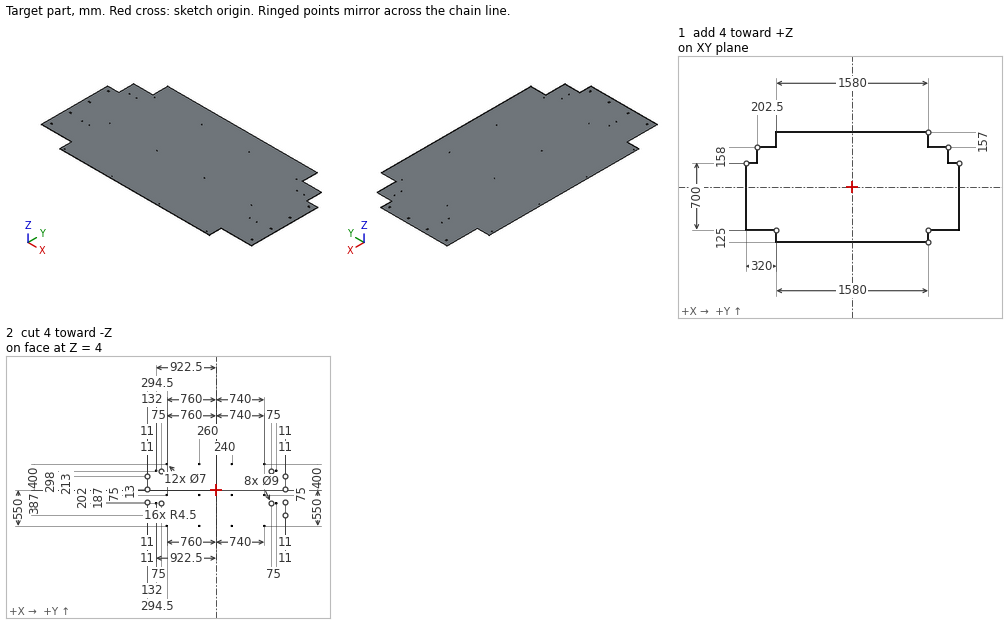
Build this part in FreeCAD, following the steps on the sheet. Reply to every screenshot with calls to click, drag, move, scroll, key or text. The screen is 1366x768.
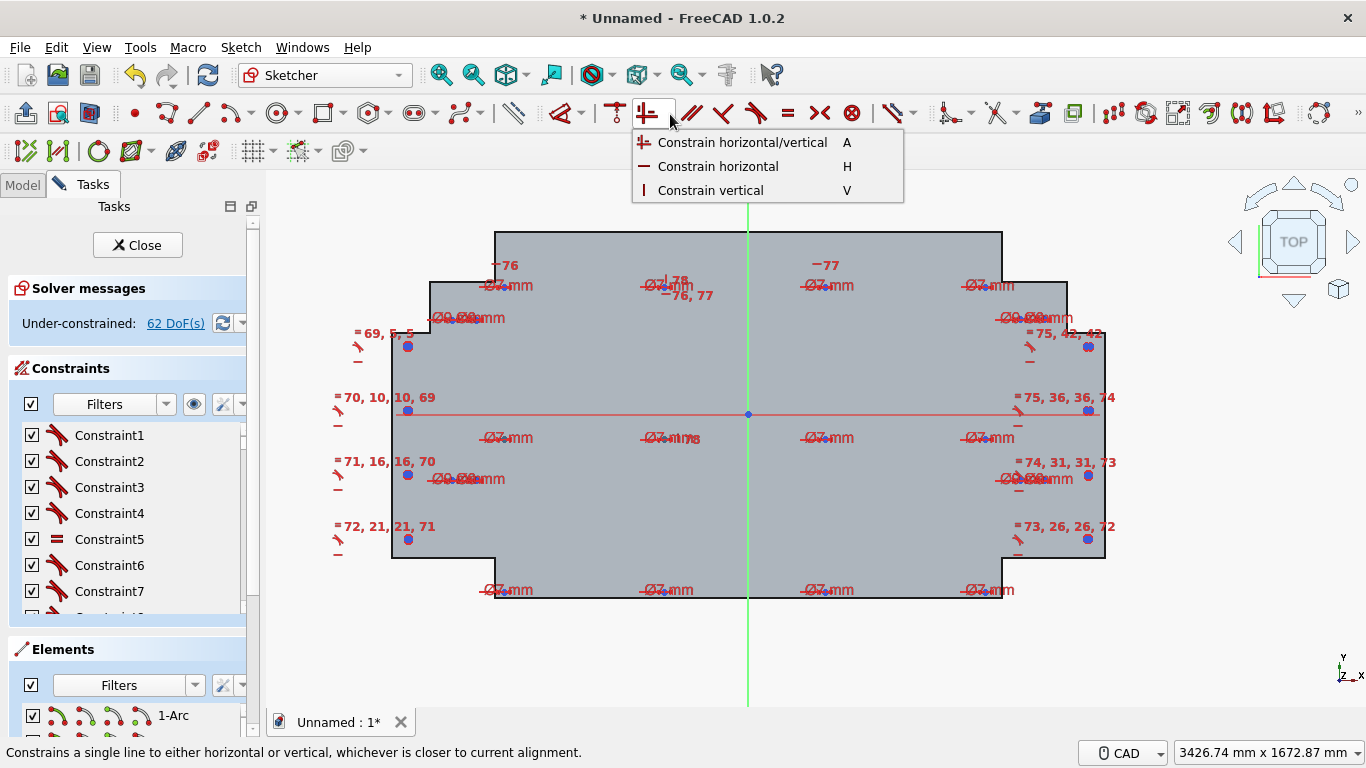
click(768, 166)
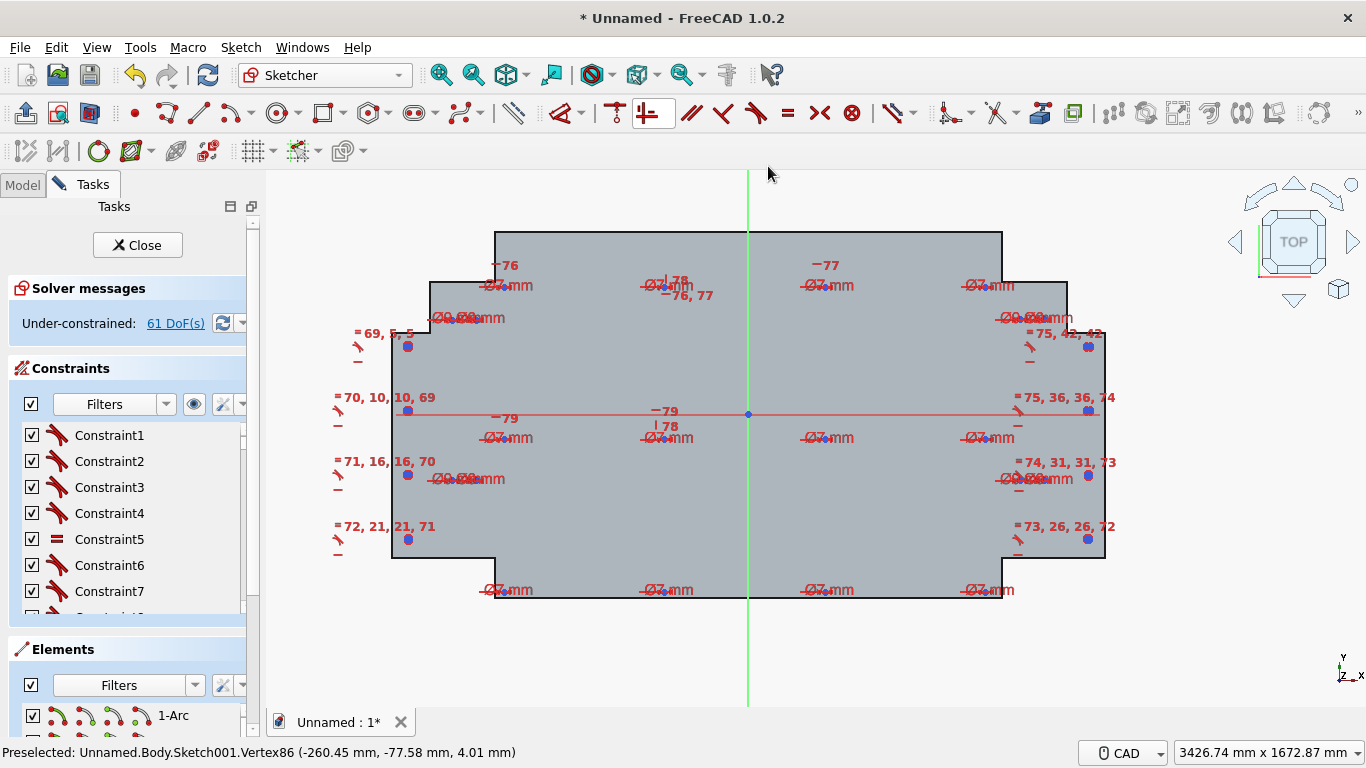
click(825, 287)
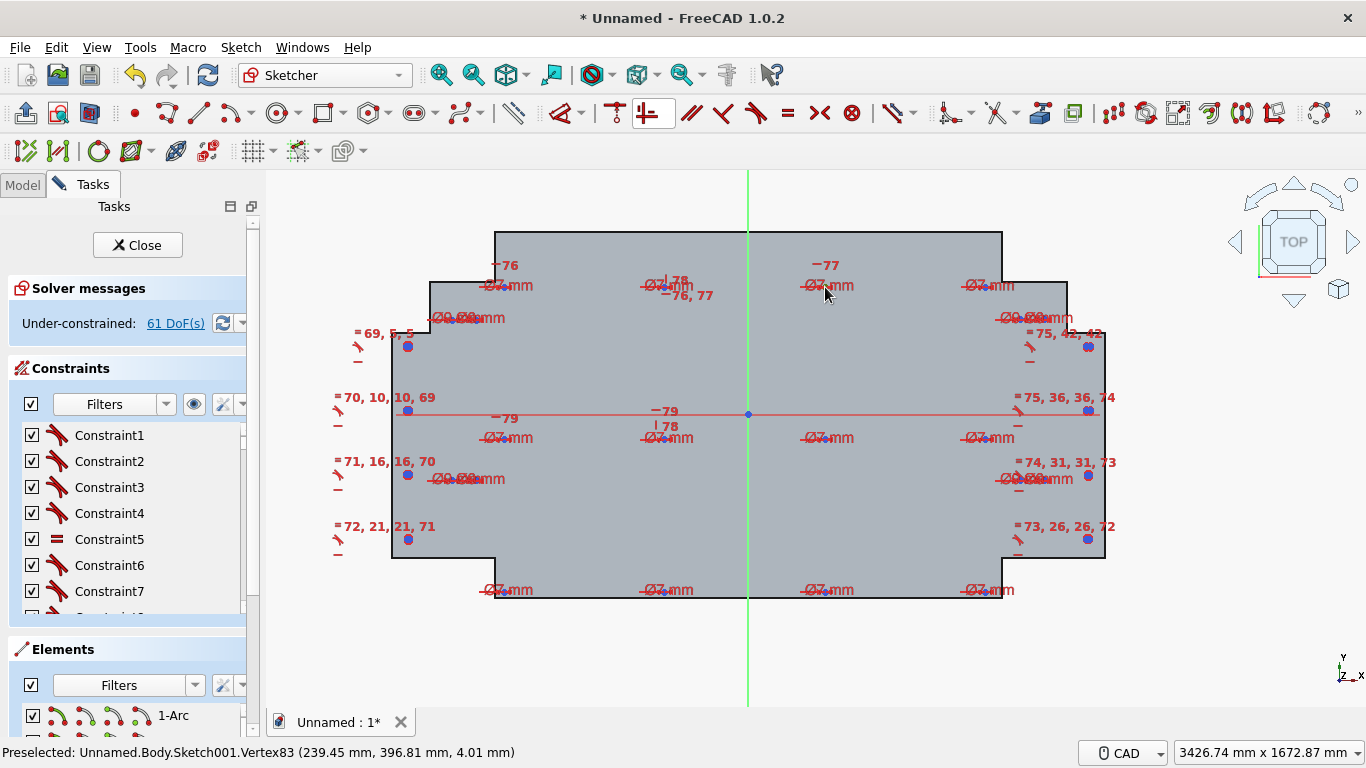
click(825, 440)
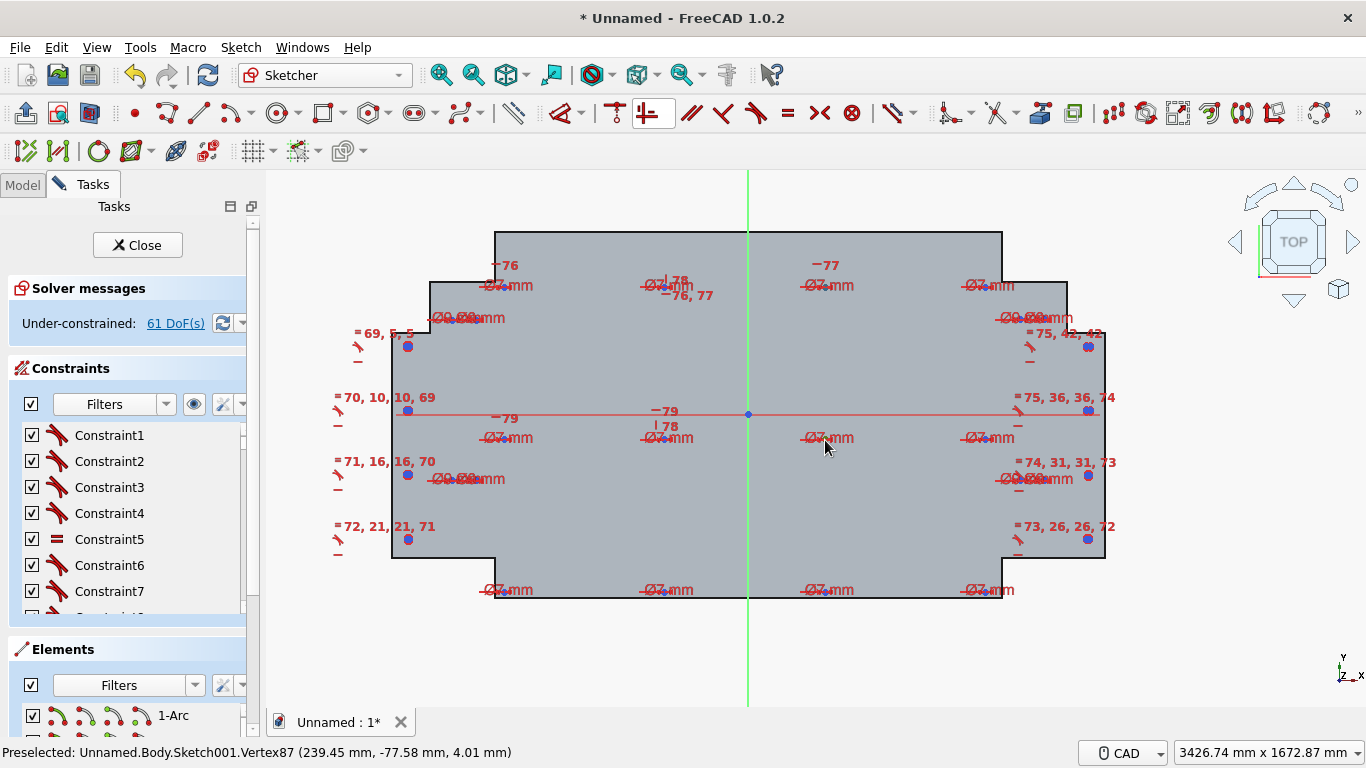
click(670, 114)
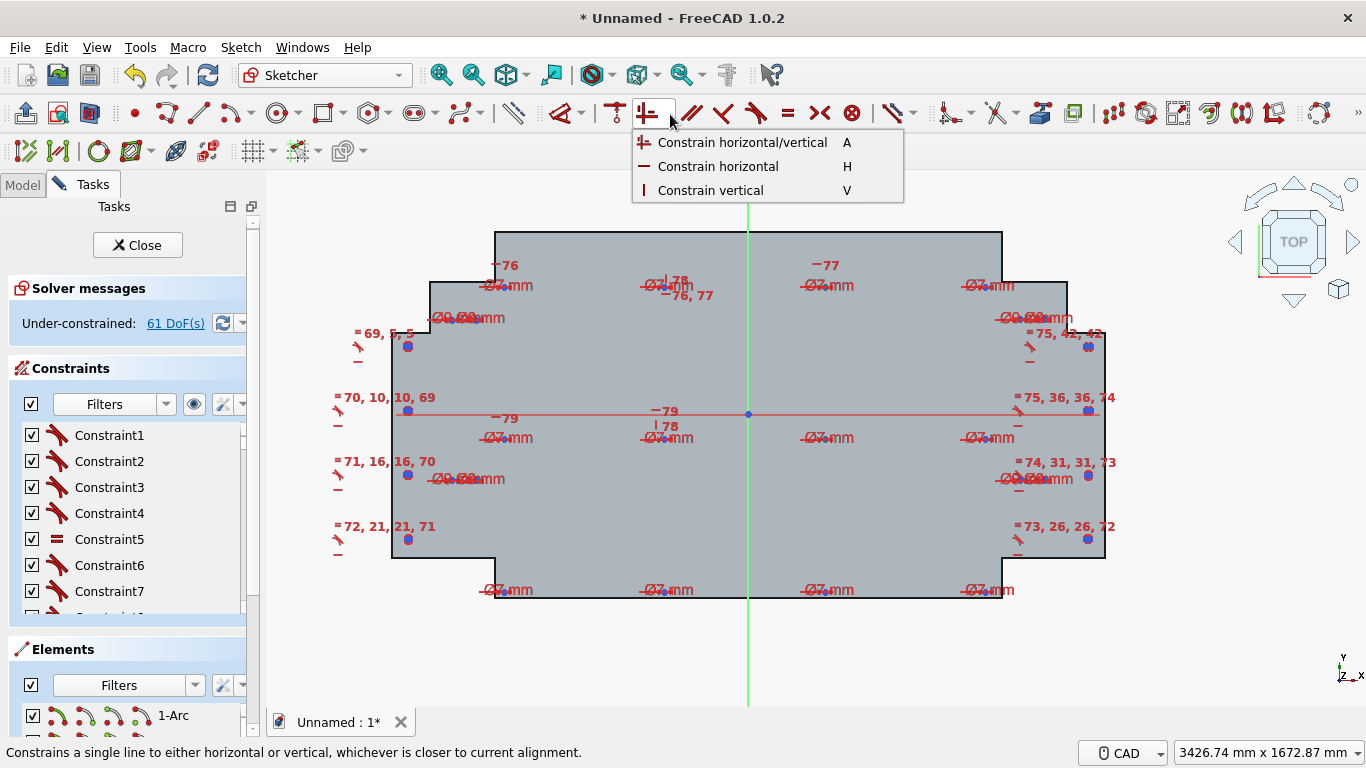
click(768, 190)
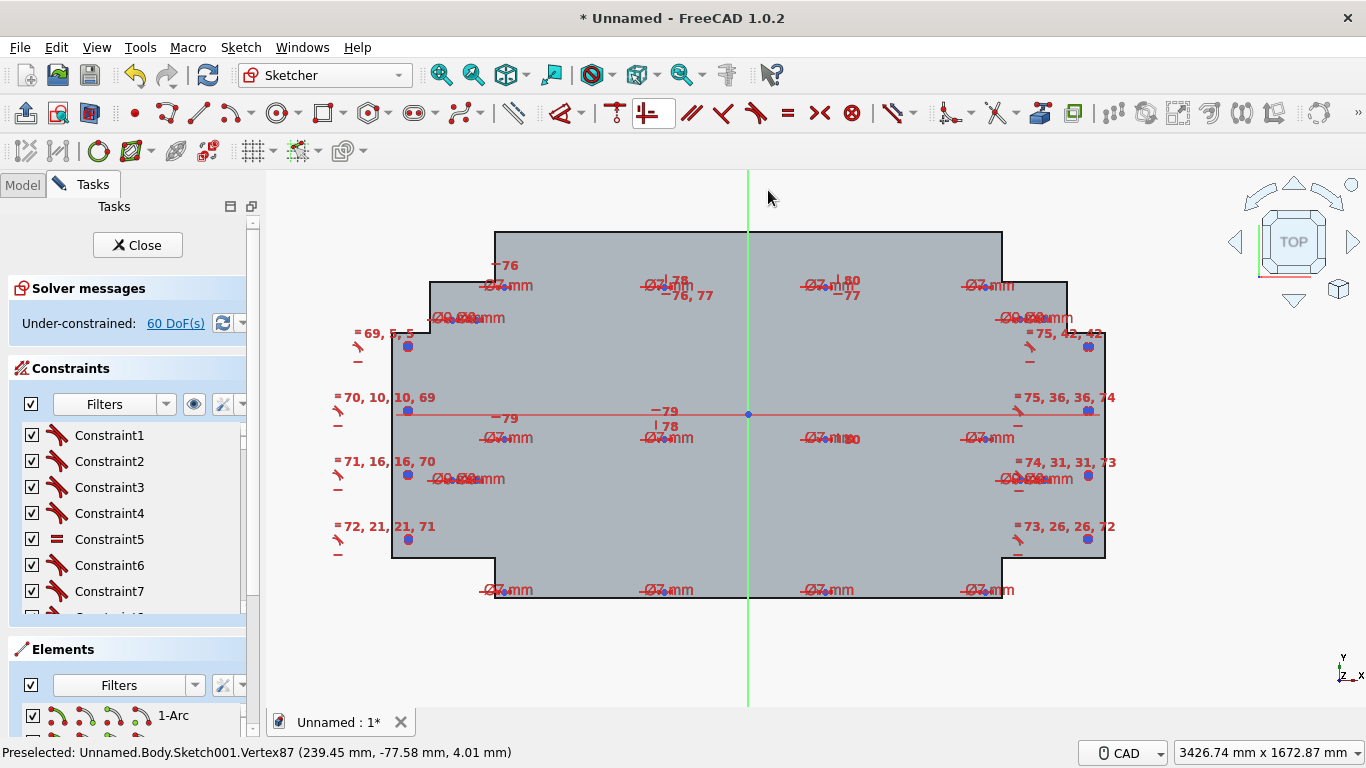
click(665, 440)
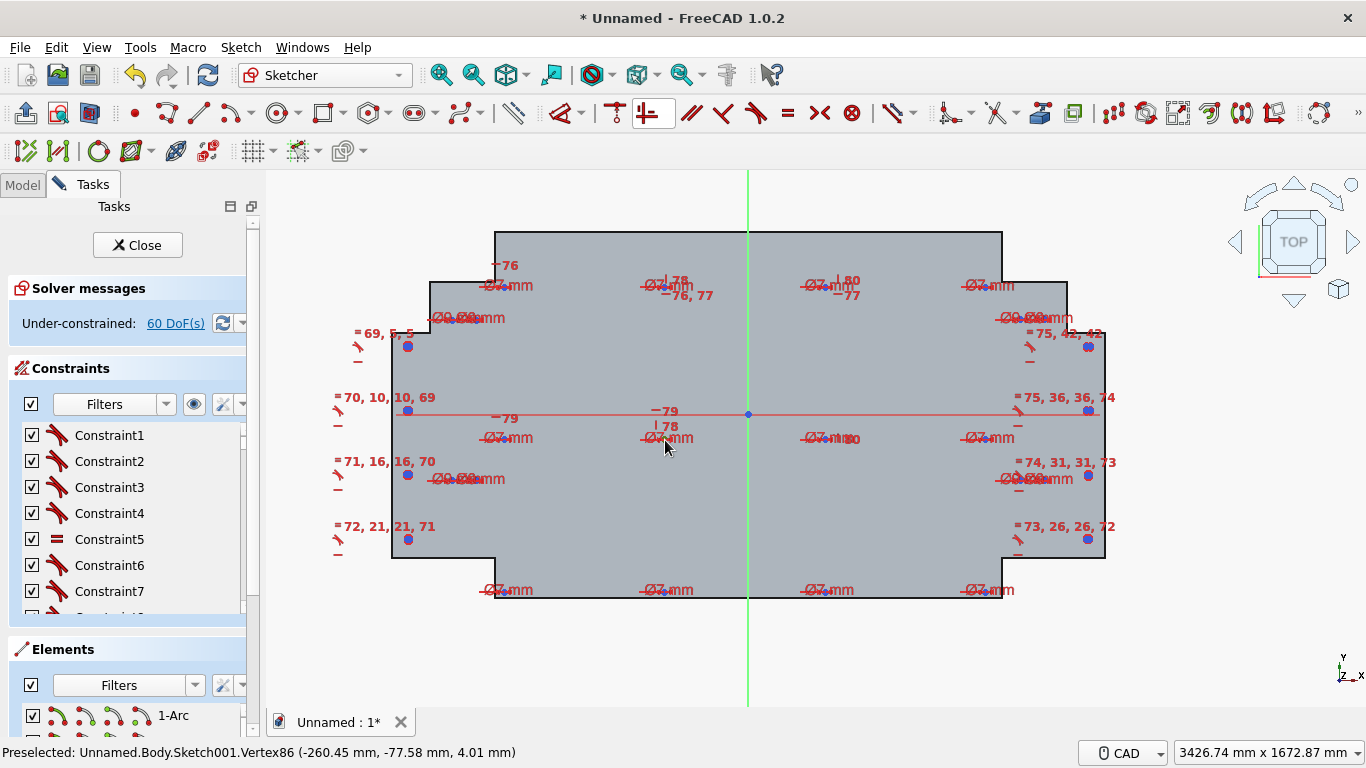
click(825, 440)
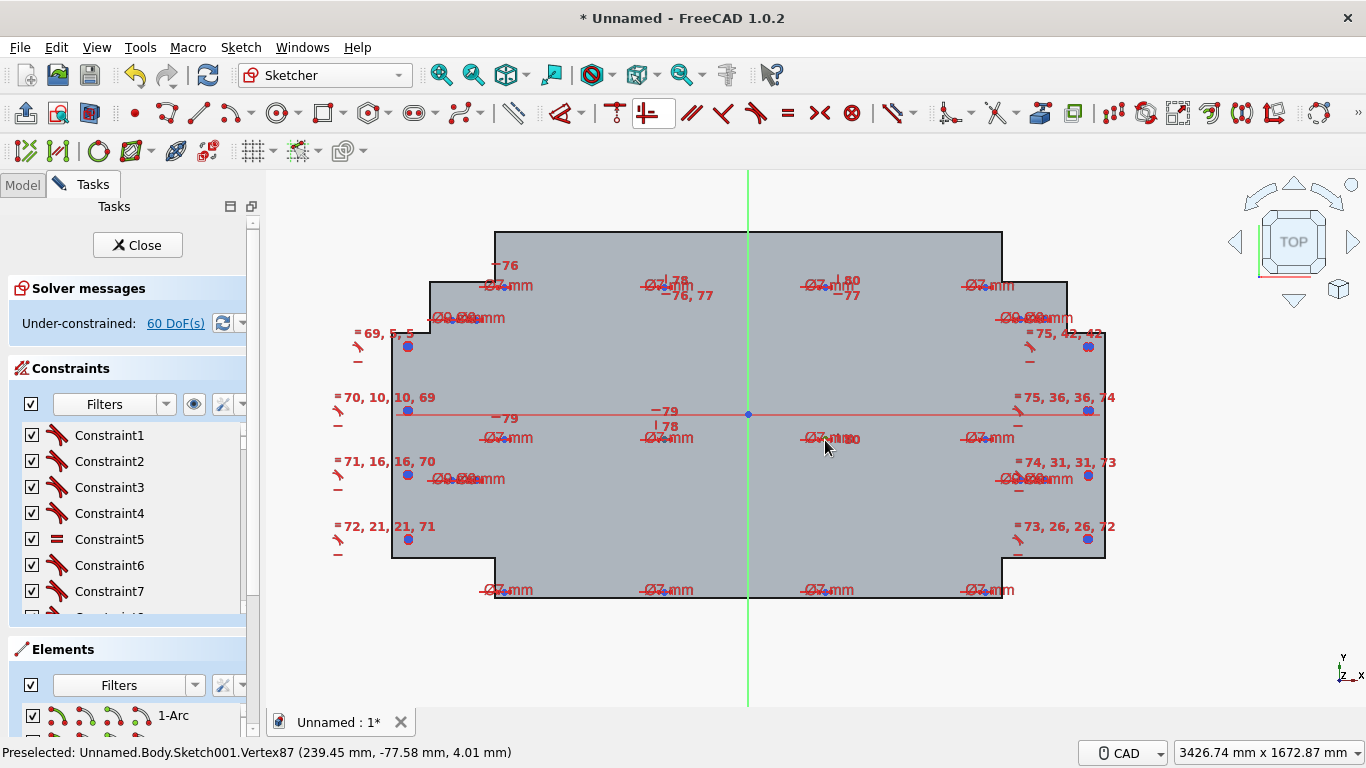
click(670, 114)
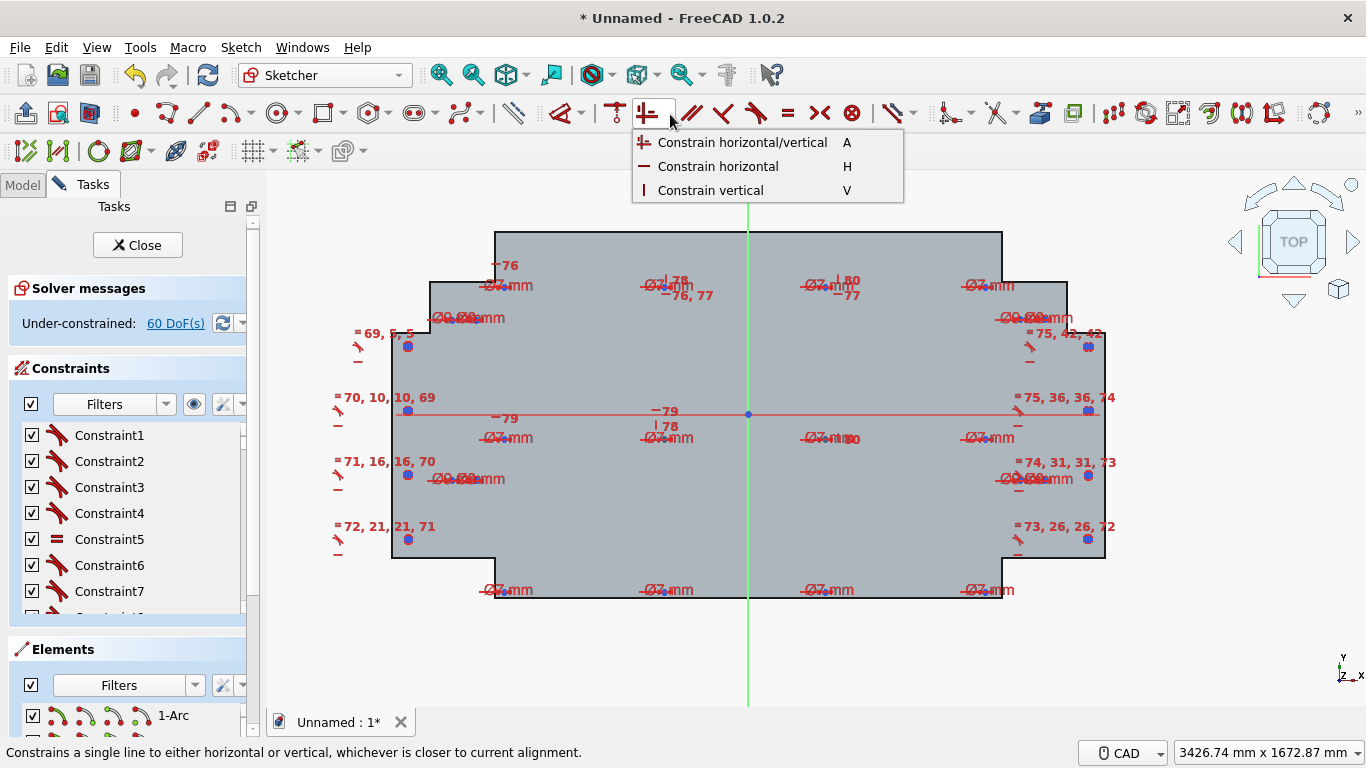
click(768, 166)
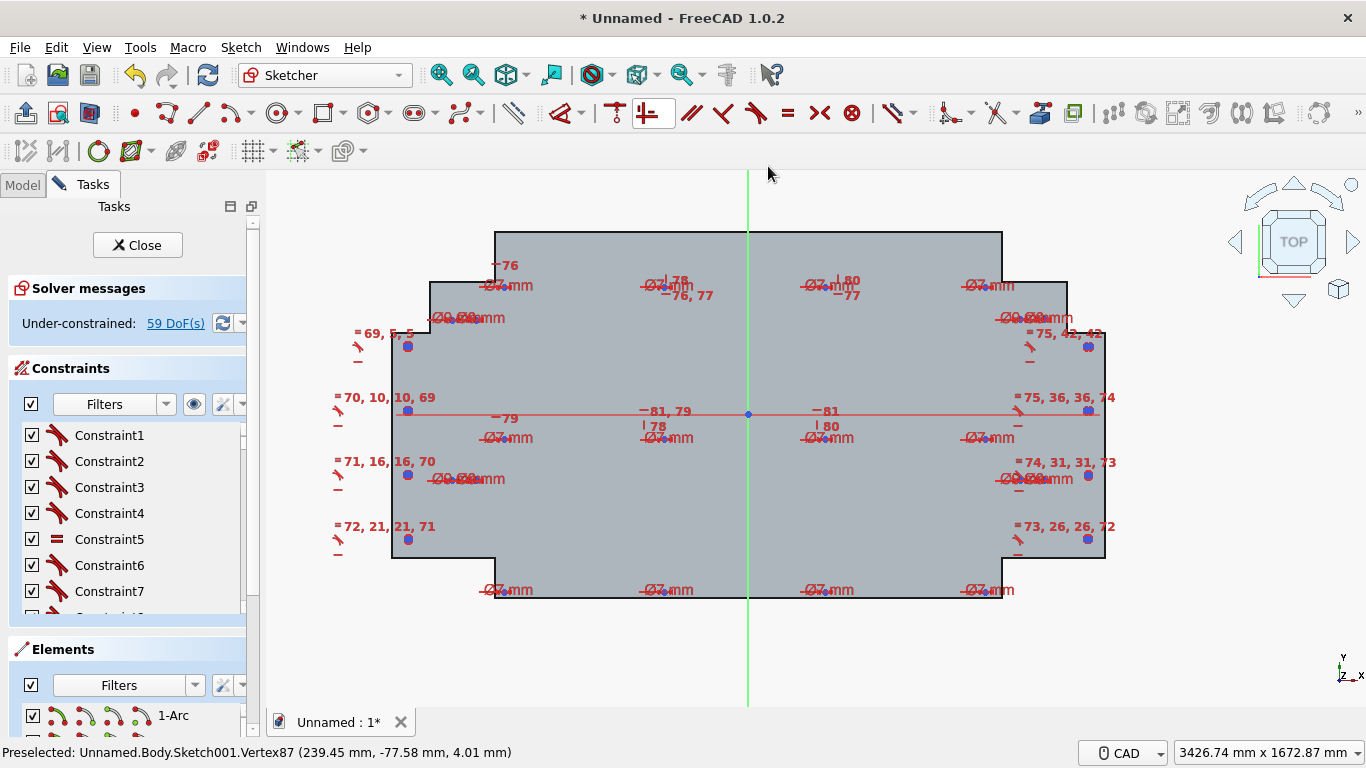
click(665, 440)